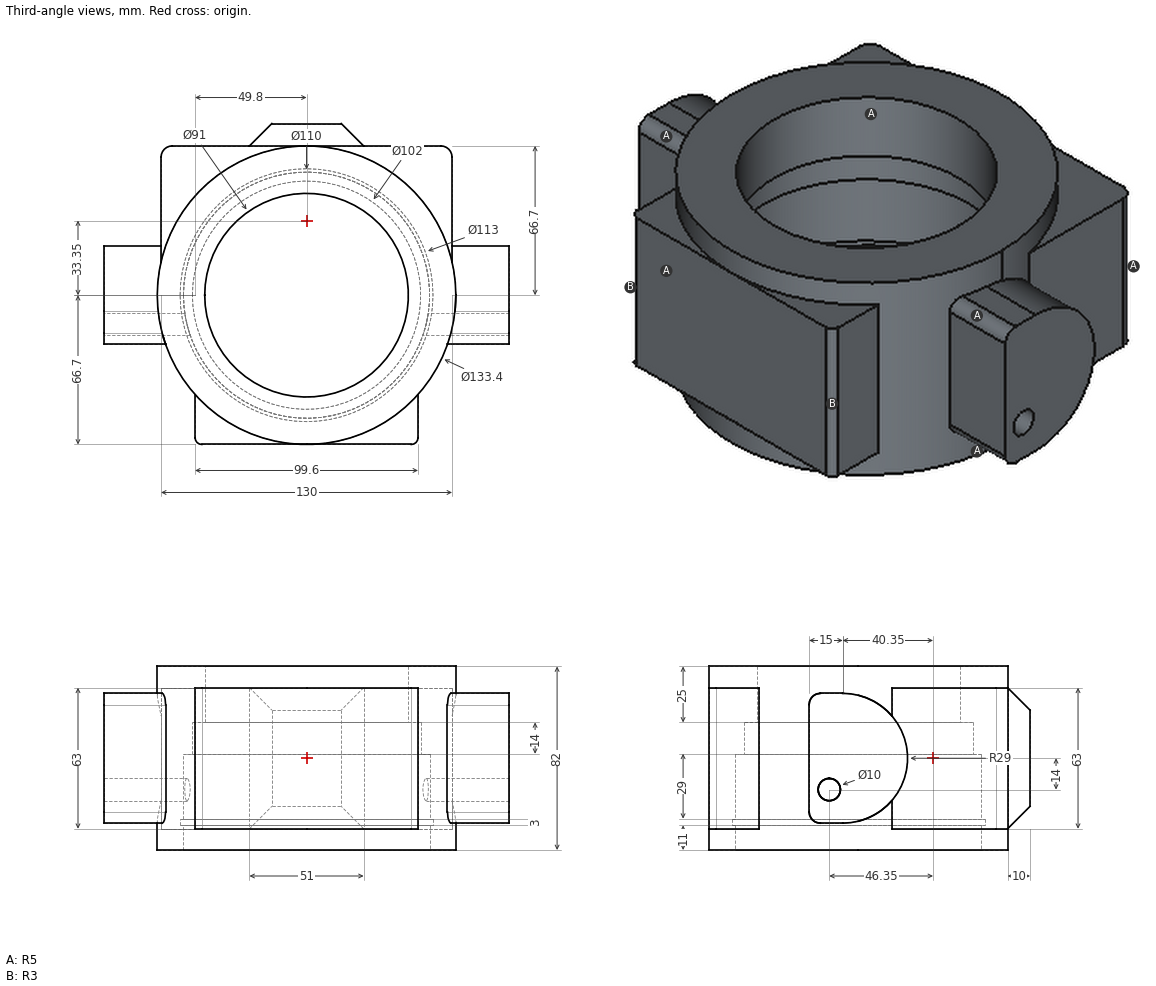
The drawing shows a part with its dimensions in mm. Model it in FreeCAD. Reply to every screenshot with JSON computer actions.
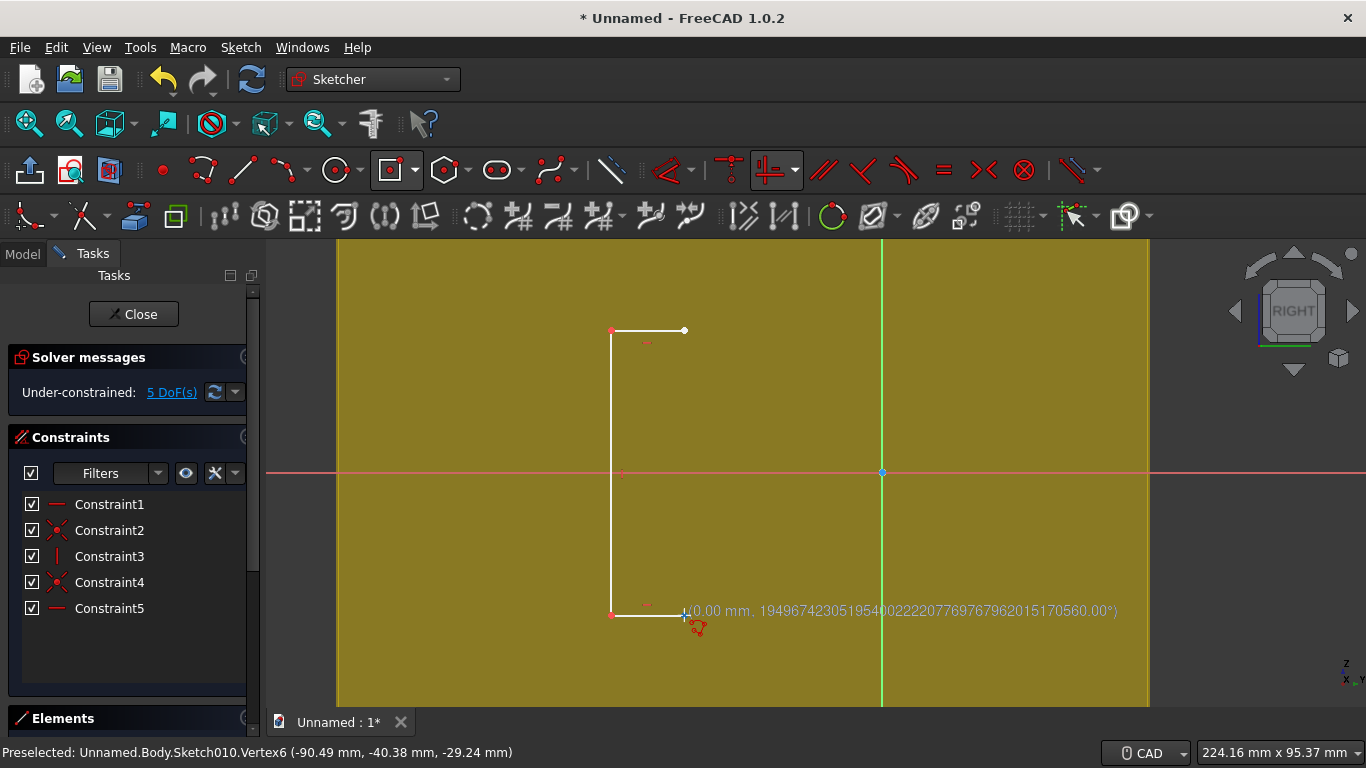
{"action": "left_click", "coordinate": [284, 170]}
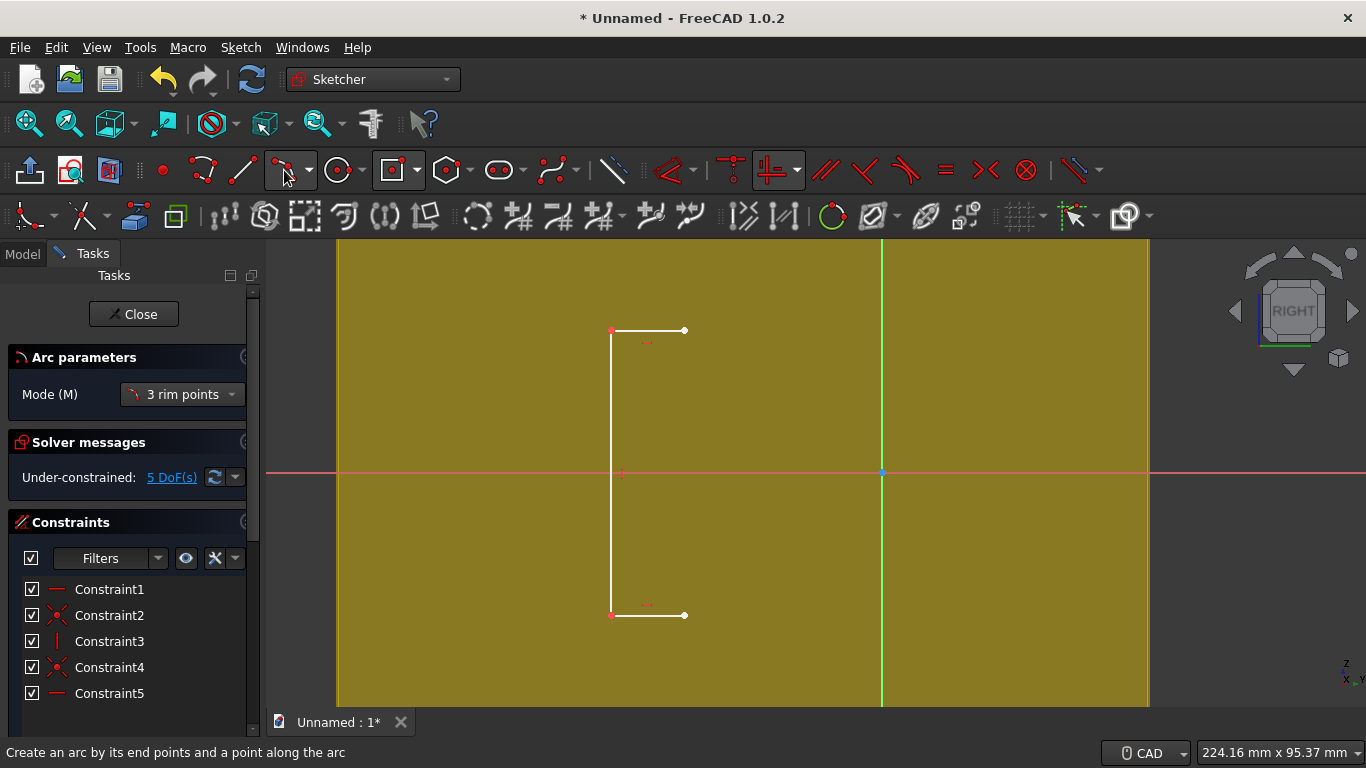
{"action": "left_click", "coordinate": [684, 616]}
{"action": "left_click", "coordinate": [684, 331]}
{"action": "left_click", "coordinate": [819, 517]}
{"action": "key", "text": "Escape"}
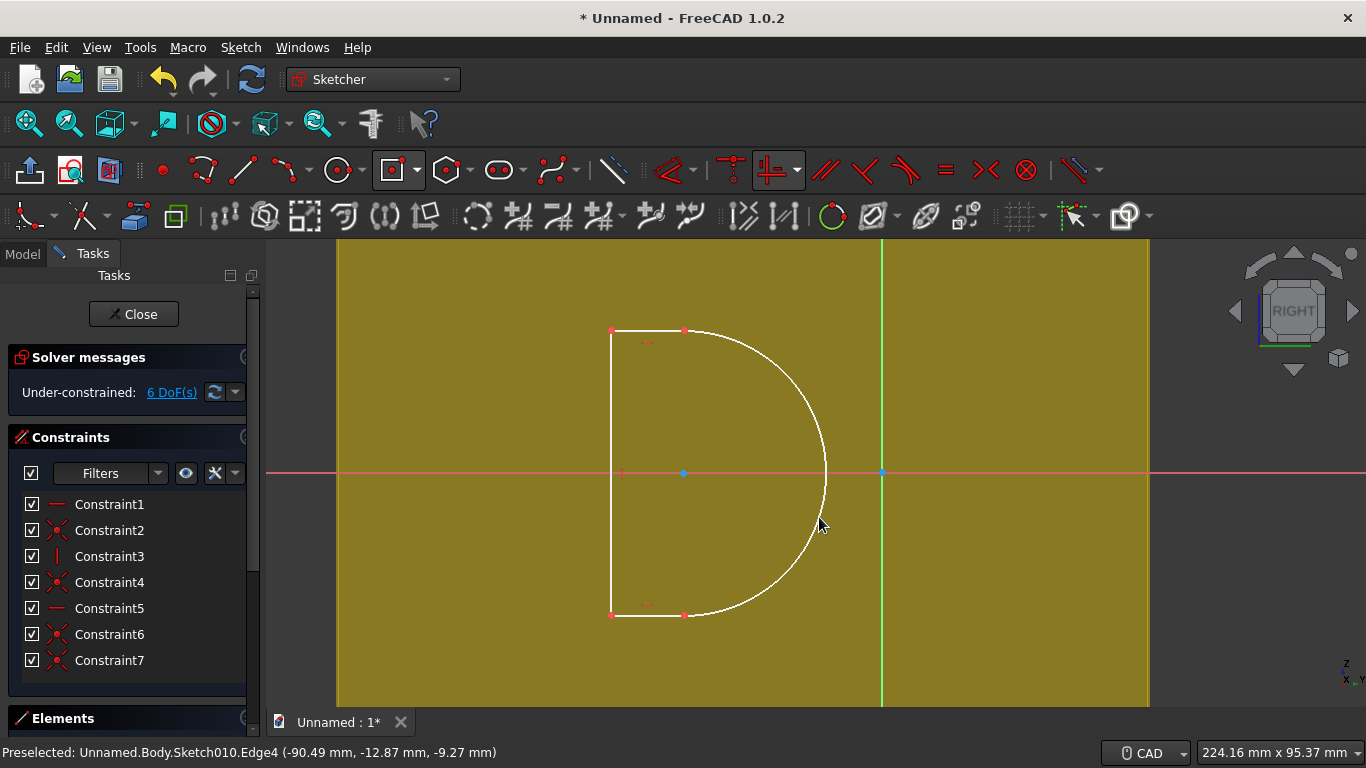
{"action": "left_click", "coordinate": [662, 331]}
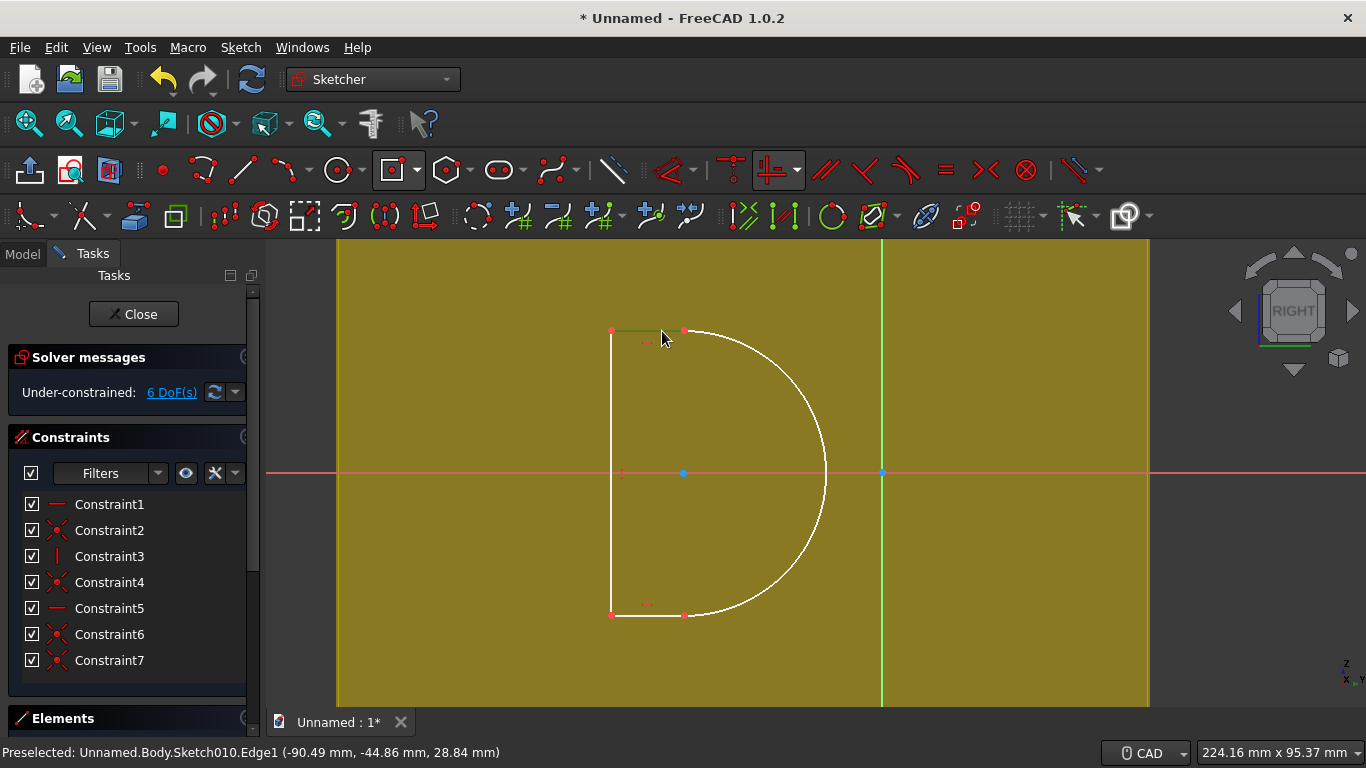
{"action": "left_click", "coordinate": [799, 557]}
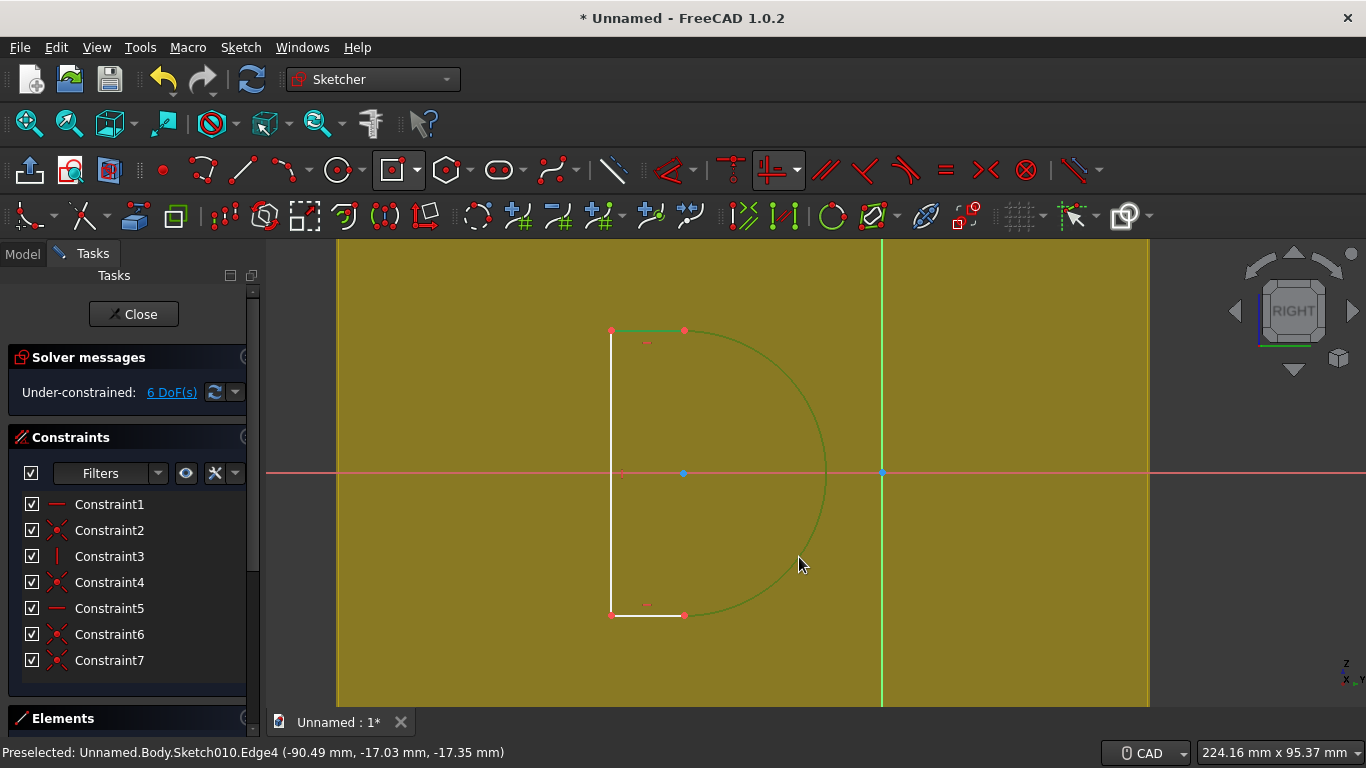
{"action": "left_click", "coordinate": [906, 170]}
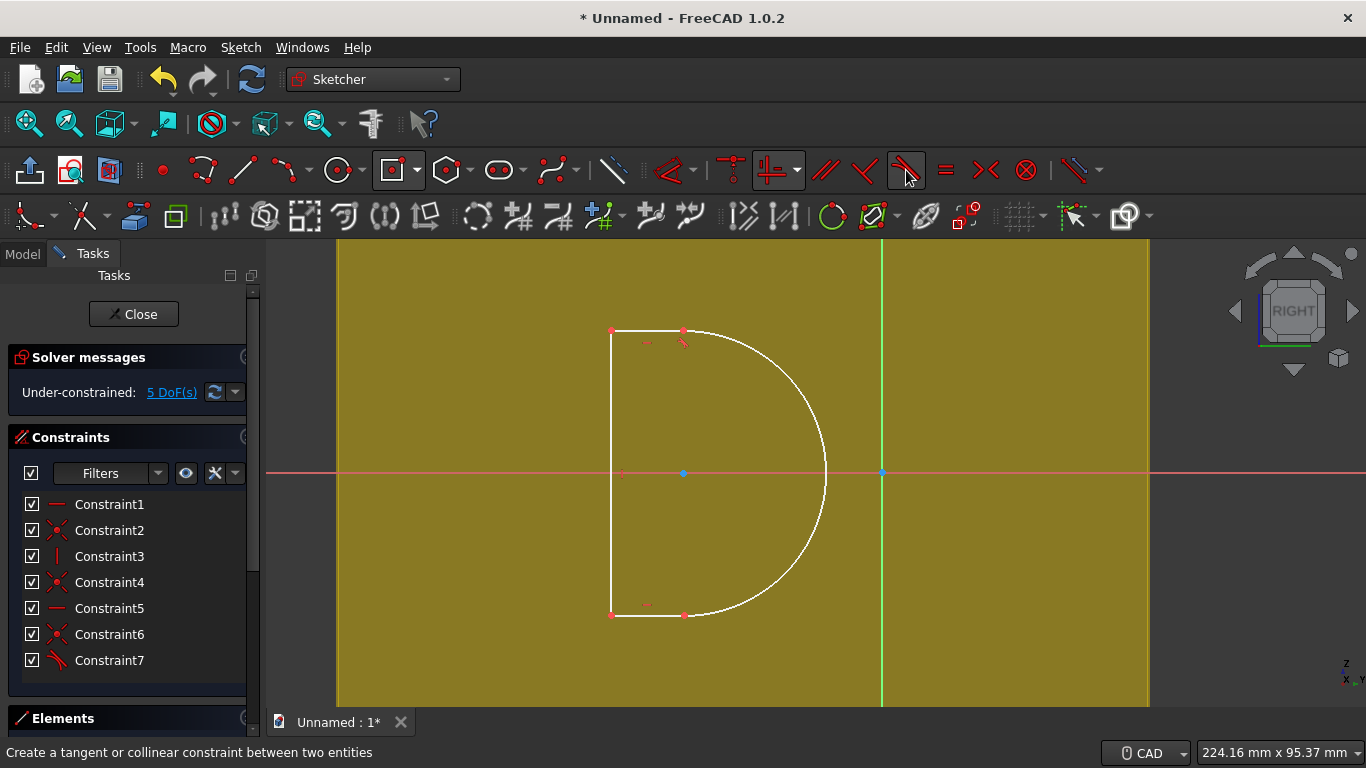
{"action": "left_click", "coordinate": [633, 616]}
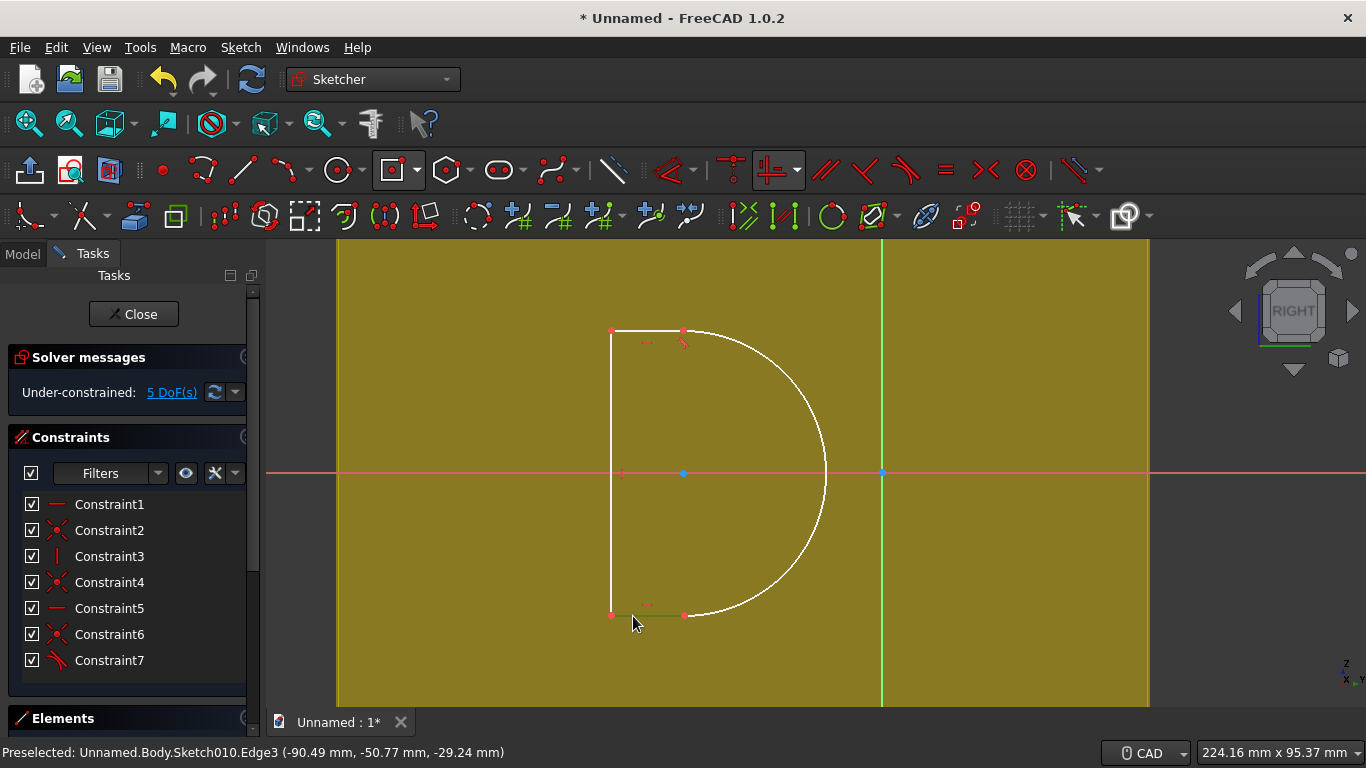
{"action": "left_click", "coordinate": [799, 557]}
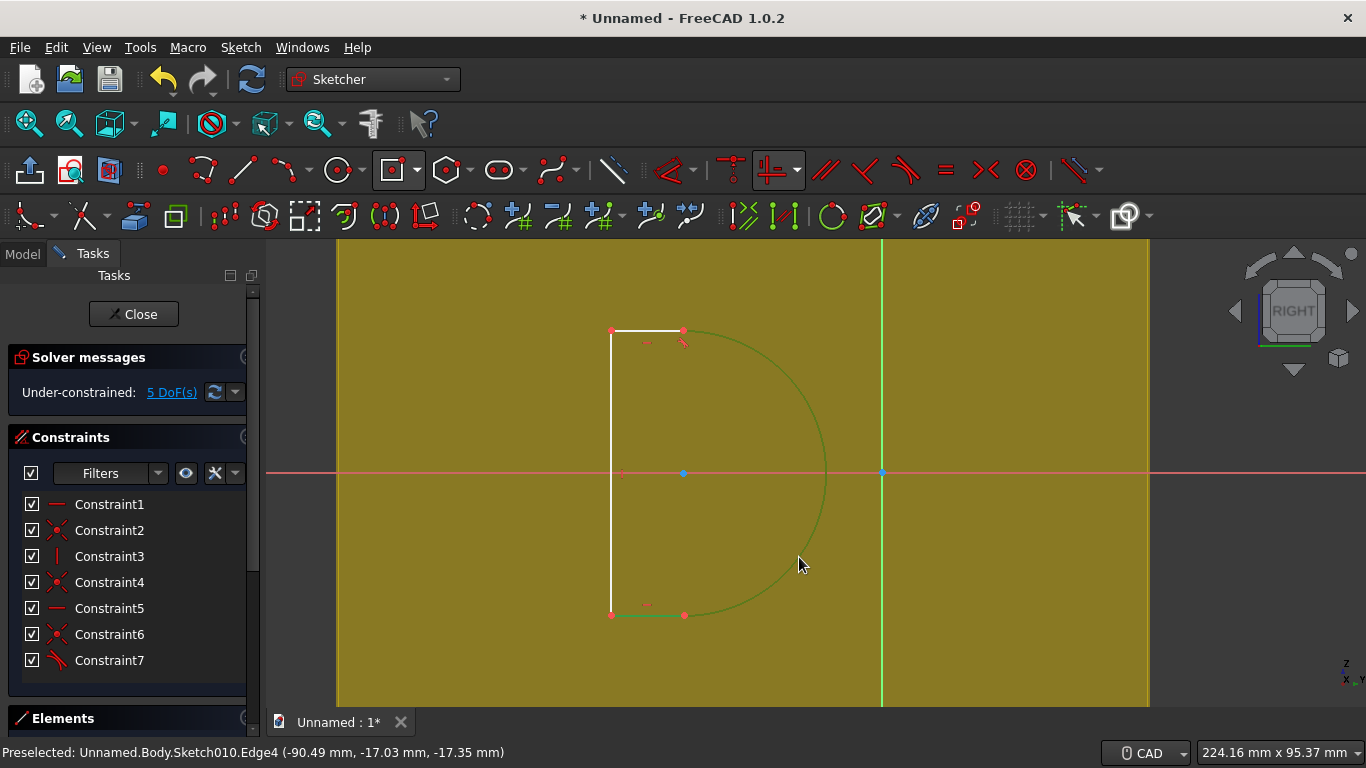
{"action": "left_click", "coordinate": [906, 170]}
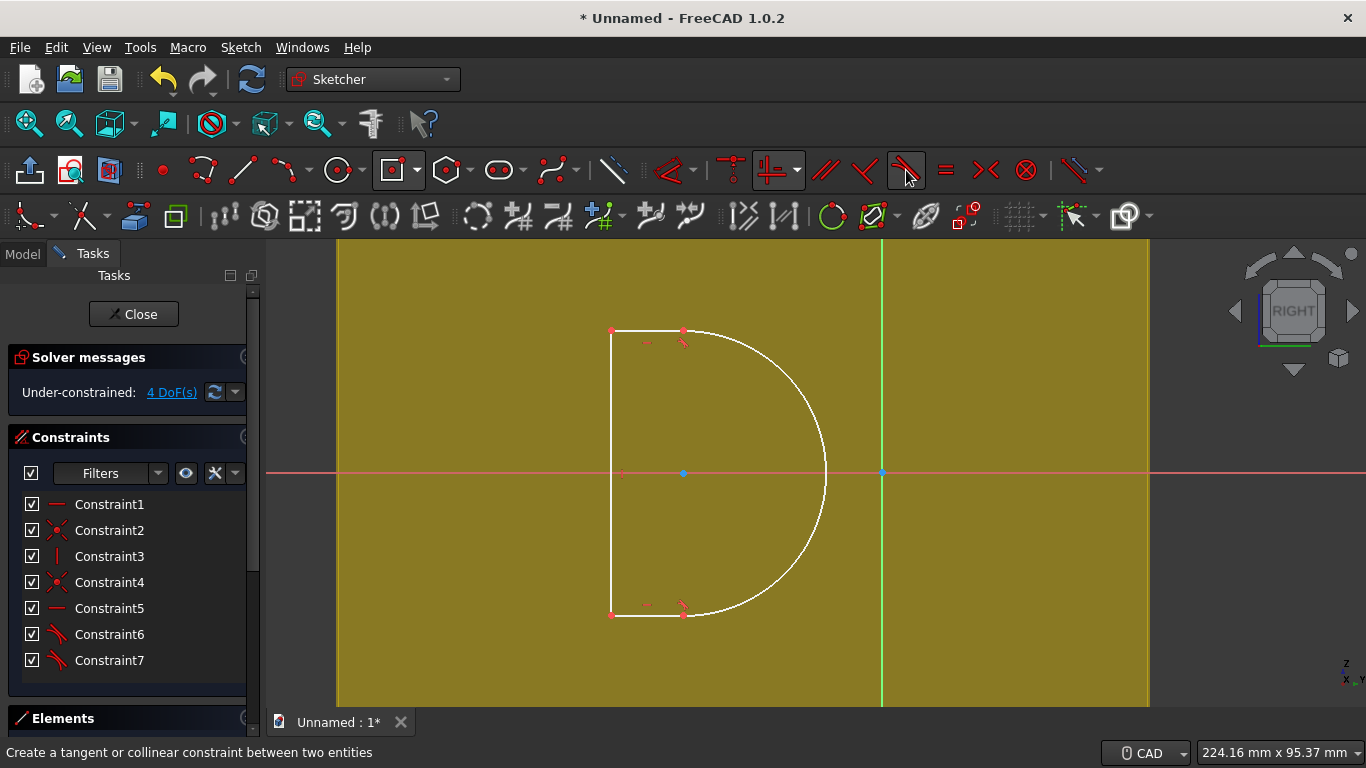
{"action": "left_click", "coordinate": [684, 473]}